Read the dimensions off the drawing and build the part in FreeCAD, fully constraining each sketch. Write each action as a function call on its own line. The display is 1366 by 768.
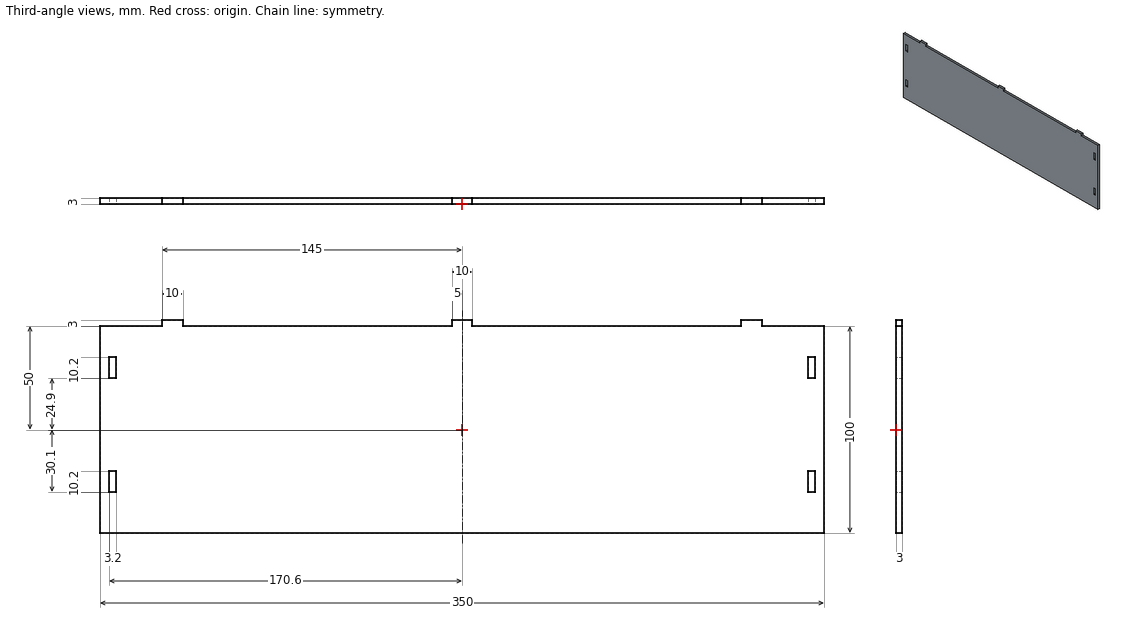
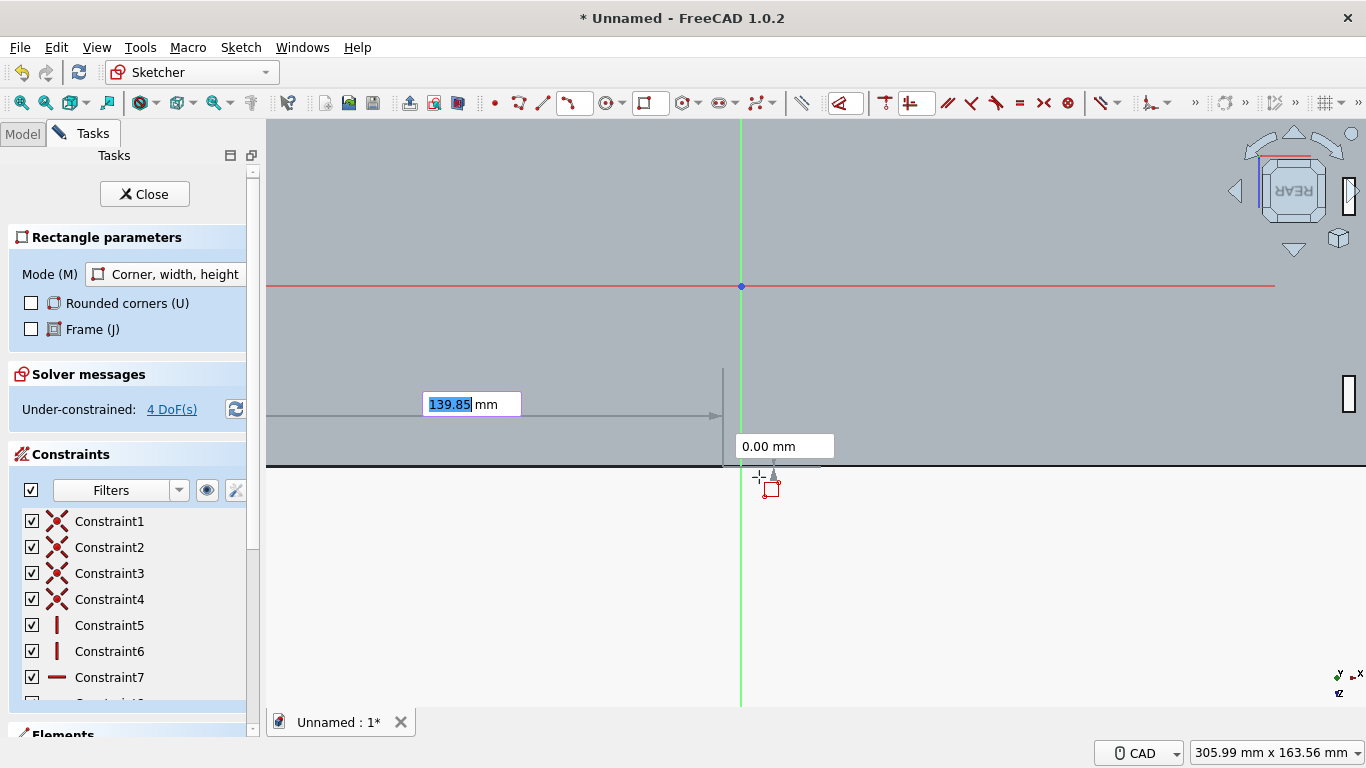
click(759, 477)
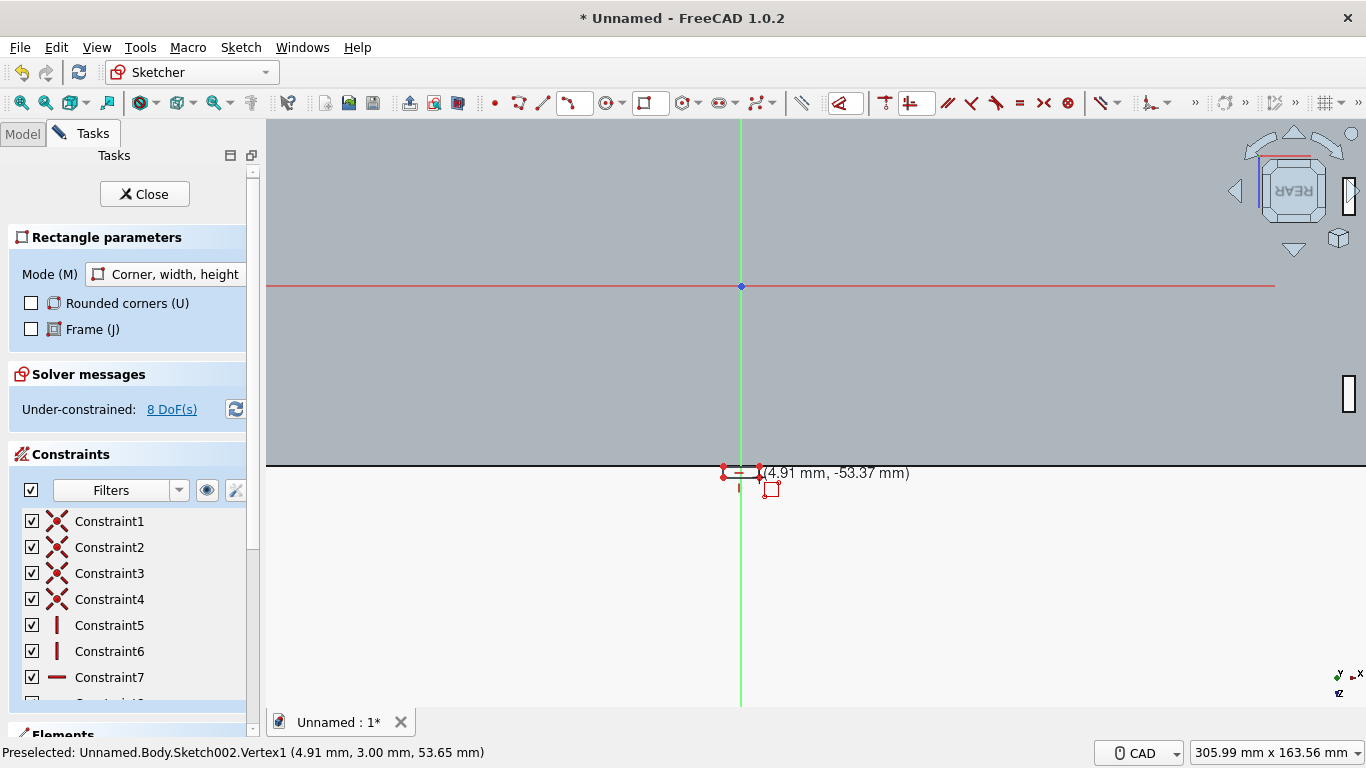
scroll(760, 477, down, 2)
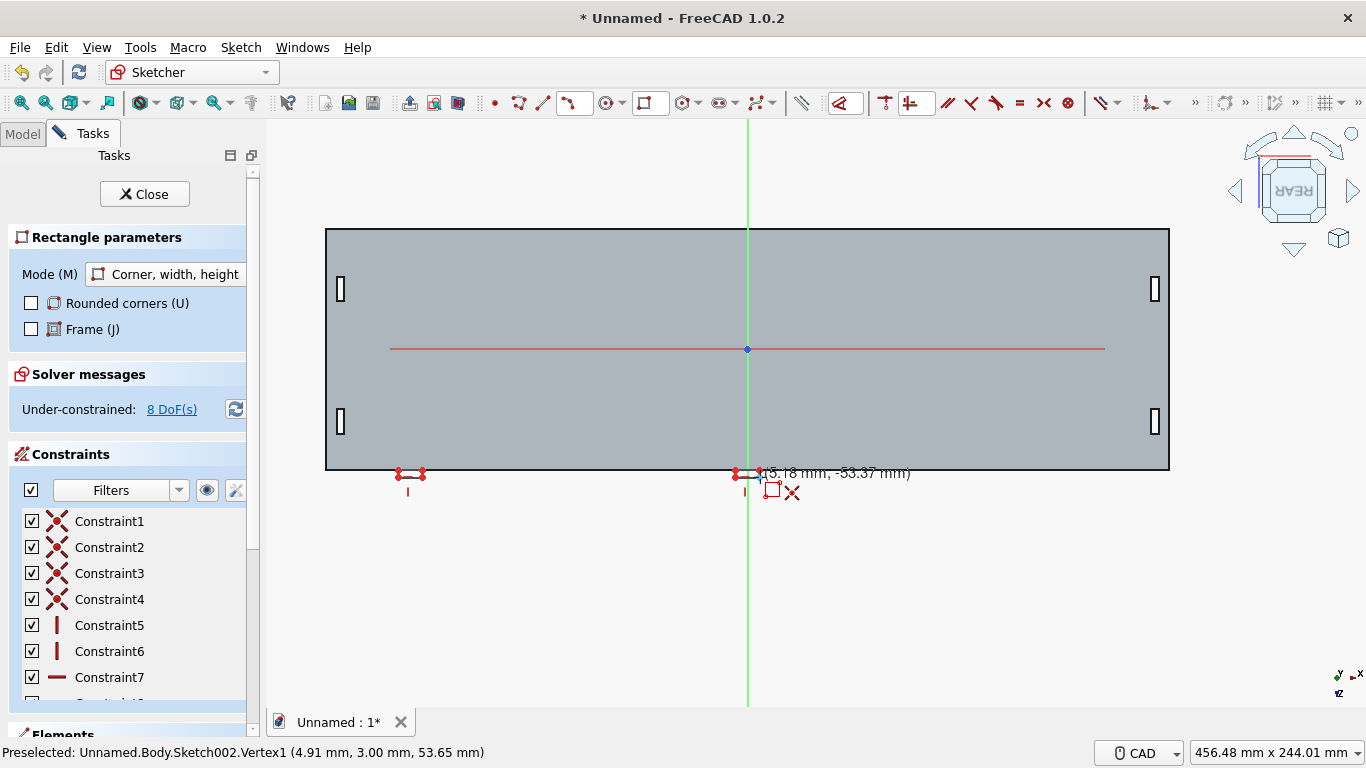
scroll(1073, 470, up, 4)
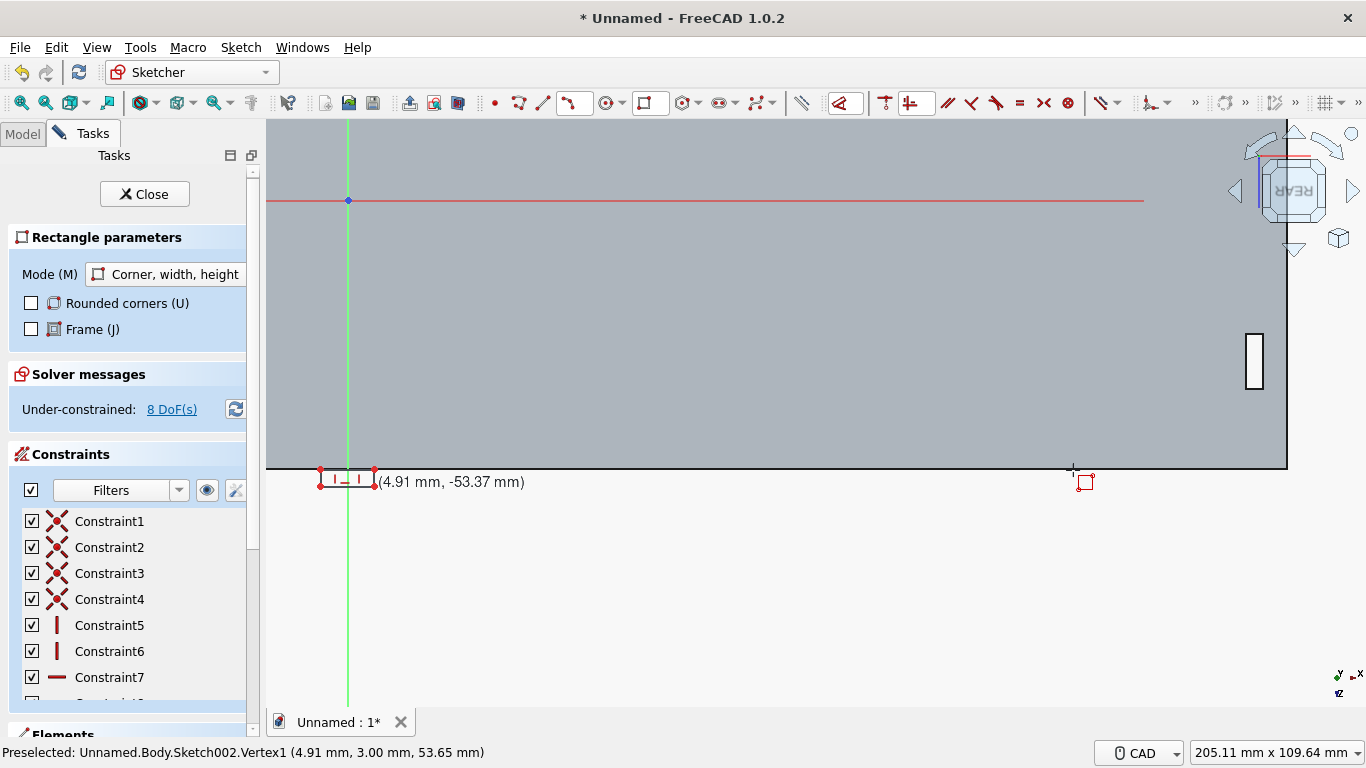
click(1072, 469)
click(1126, 485)
key(Escape)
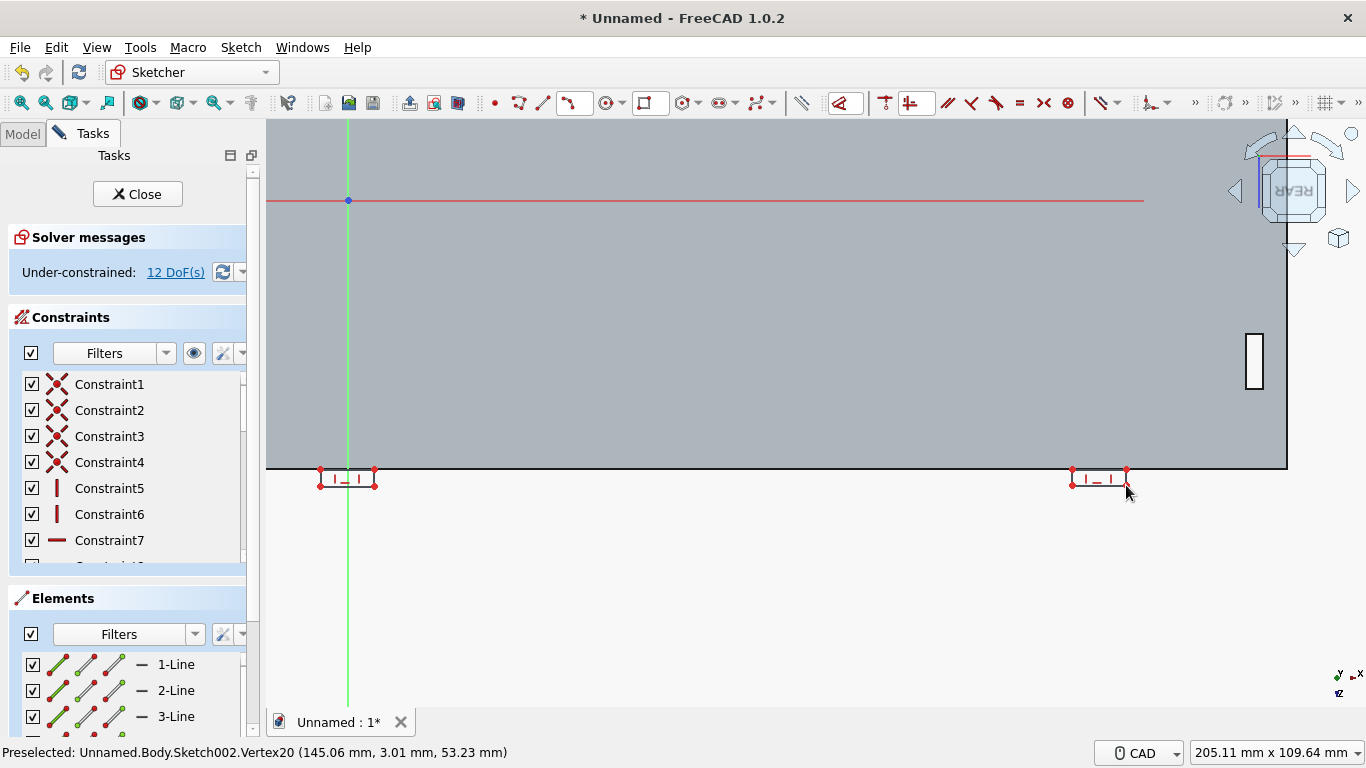
scroll(1073, 470, down, 4)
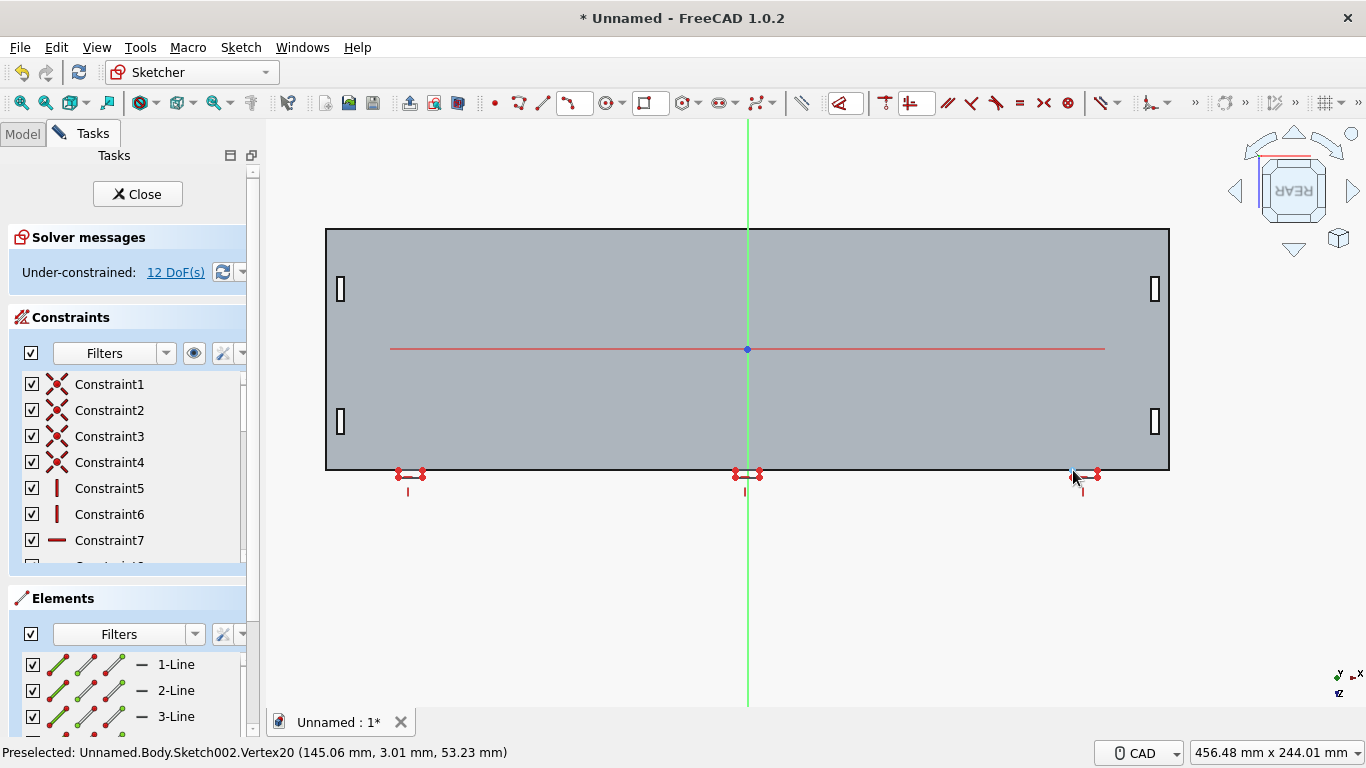
scroll(422, 470, up, 3)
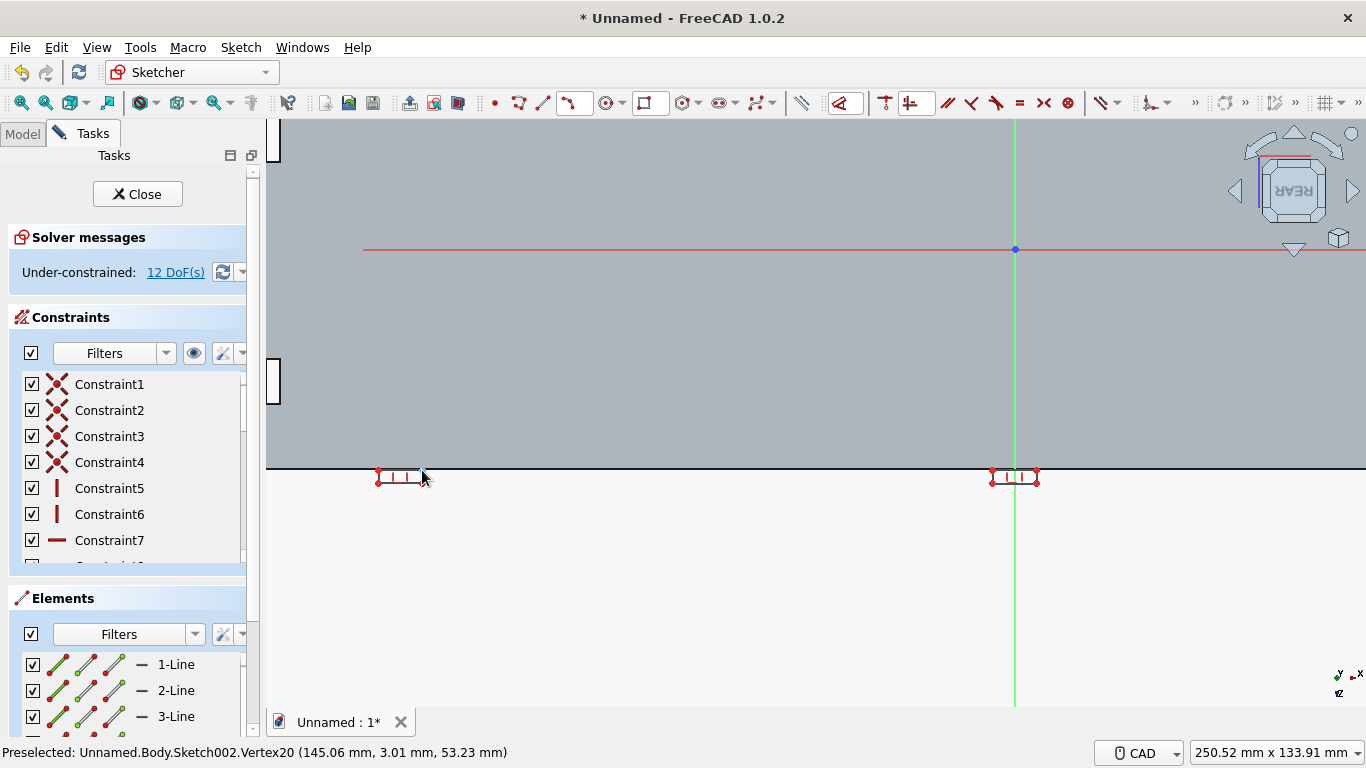
click(422, 470)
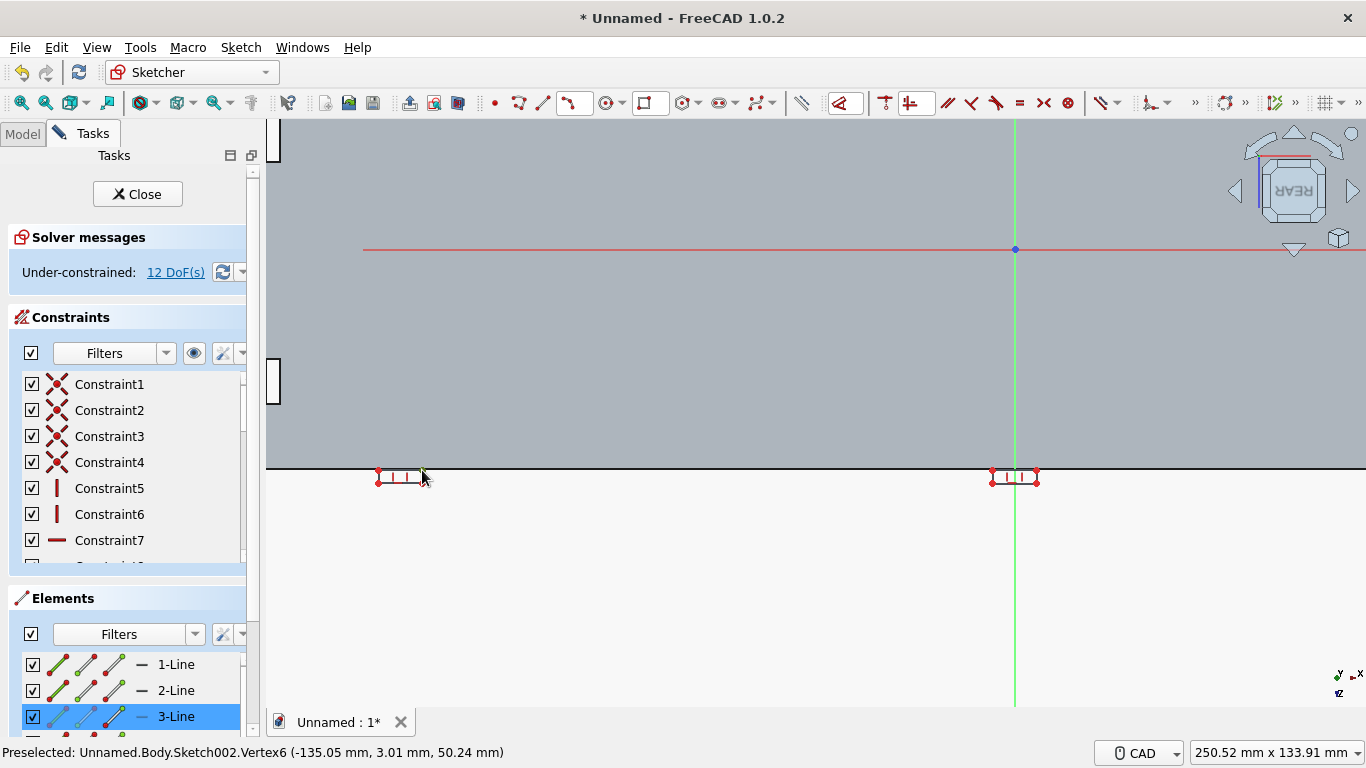
scroll(422, 470, down, 3)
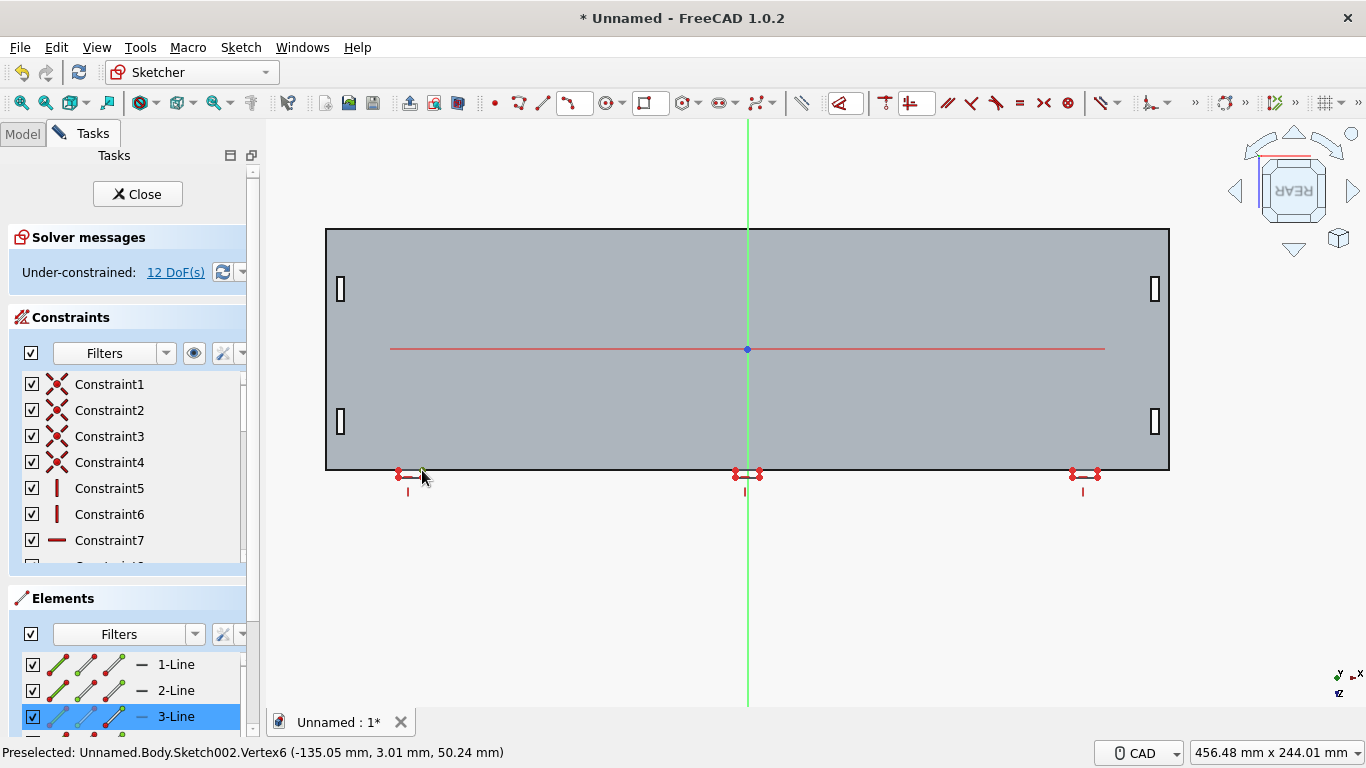
scroll(1073, 470, up, 3)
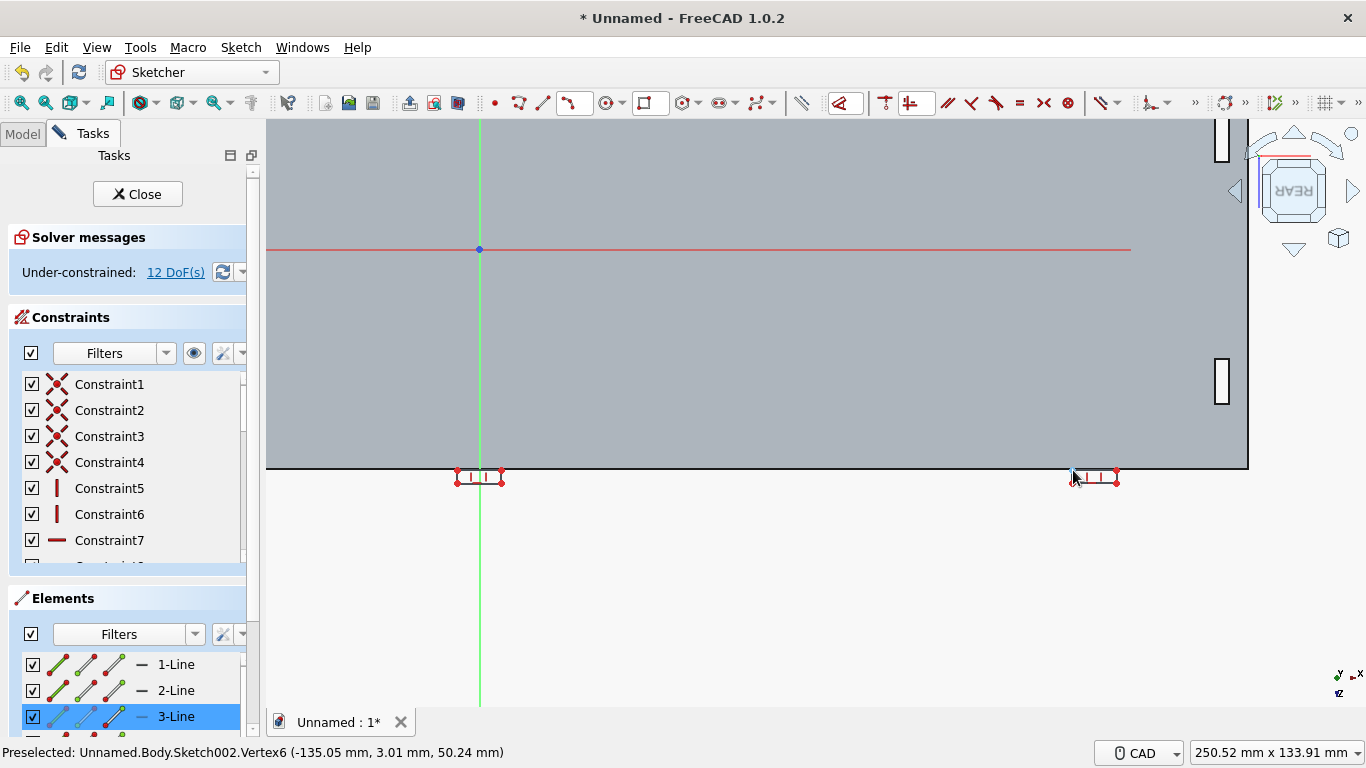
click(1072, 470)